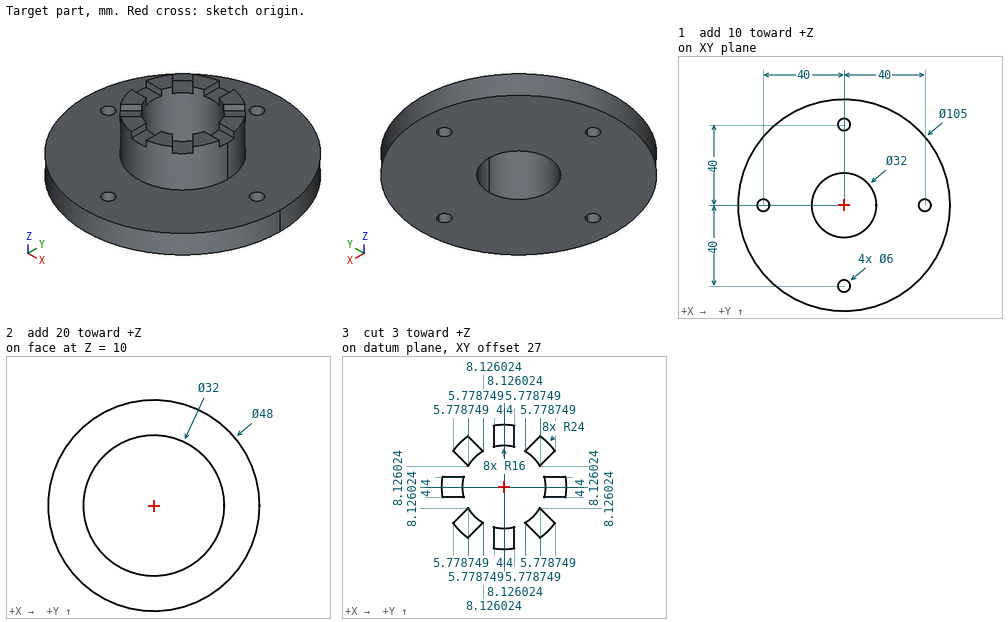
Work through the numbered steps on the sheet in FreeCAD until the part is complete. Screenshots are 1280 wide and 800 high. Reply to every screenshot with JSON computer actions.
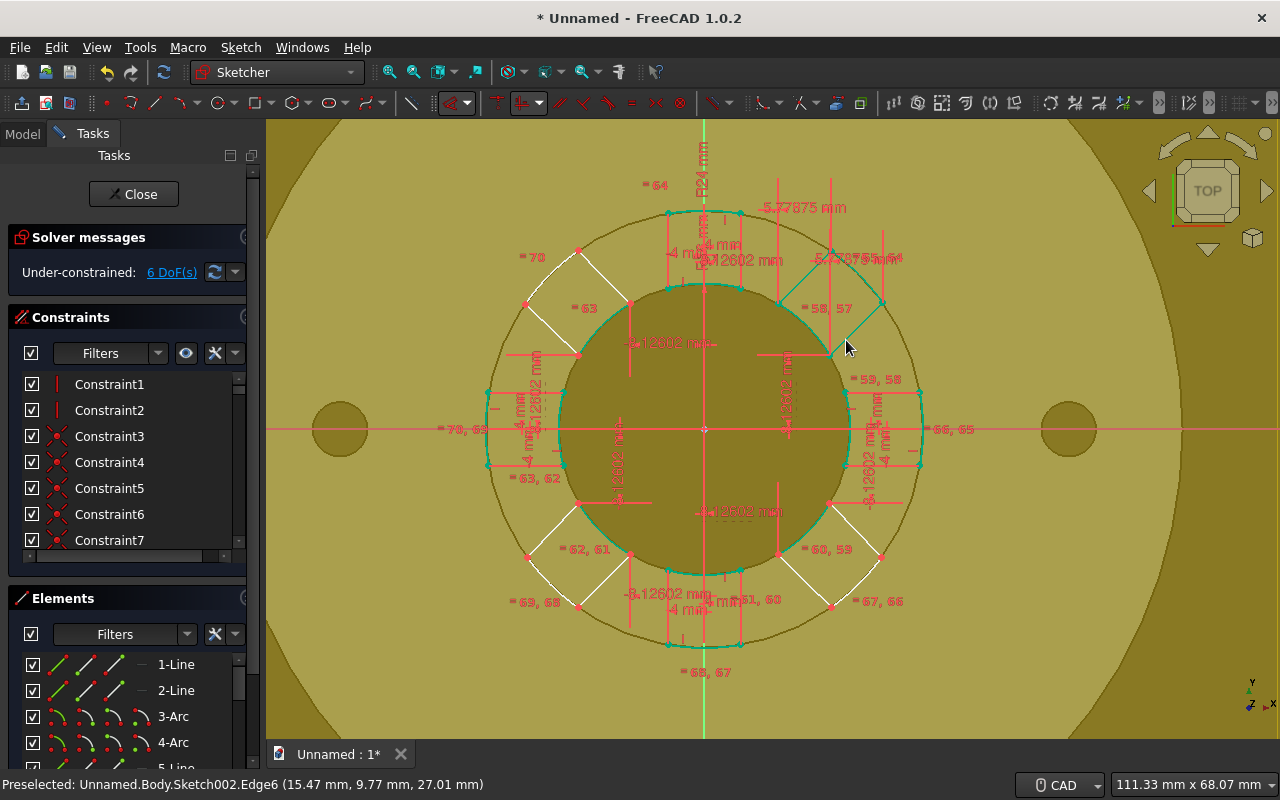
{"action": "left_click", "coordinate": [866, 541]}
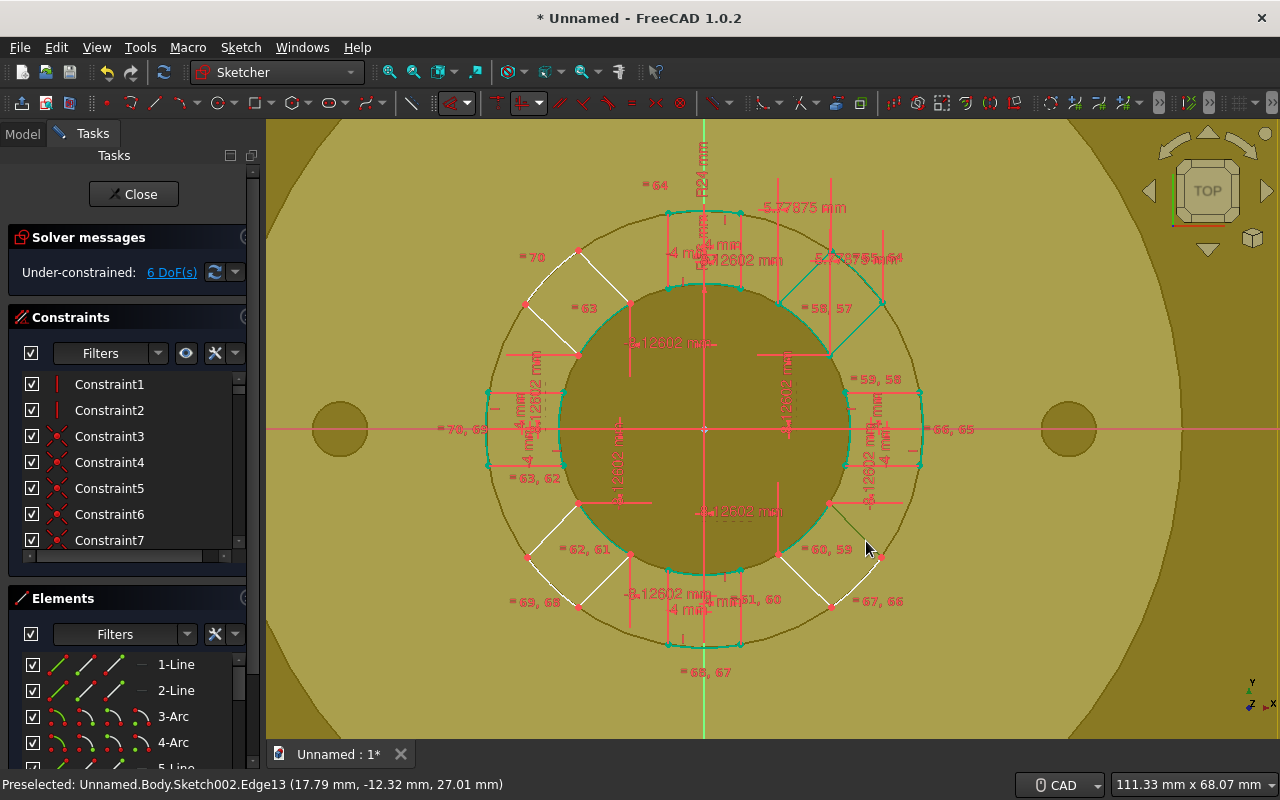
{"action": "key", "text": "l"}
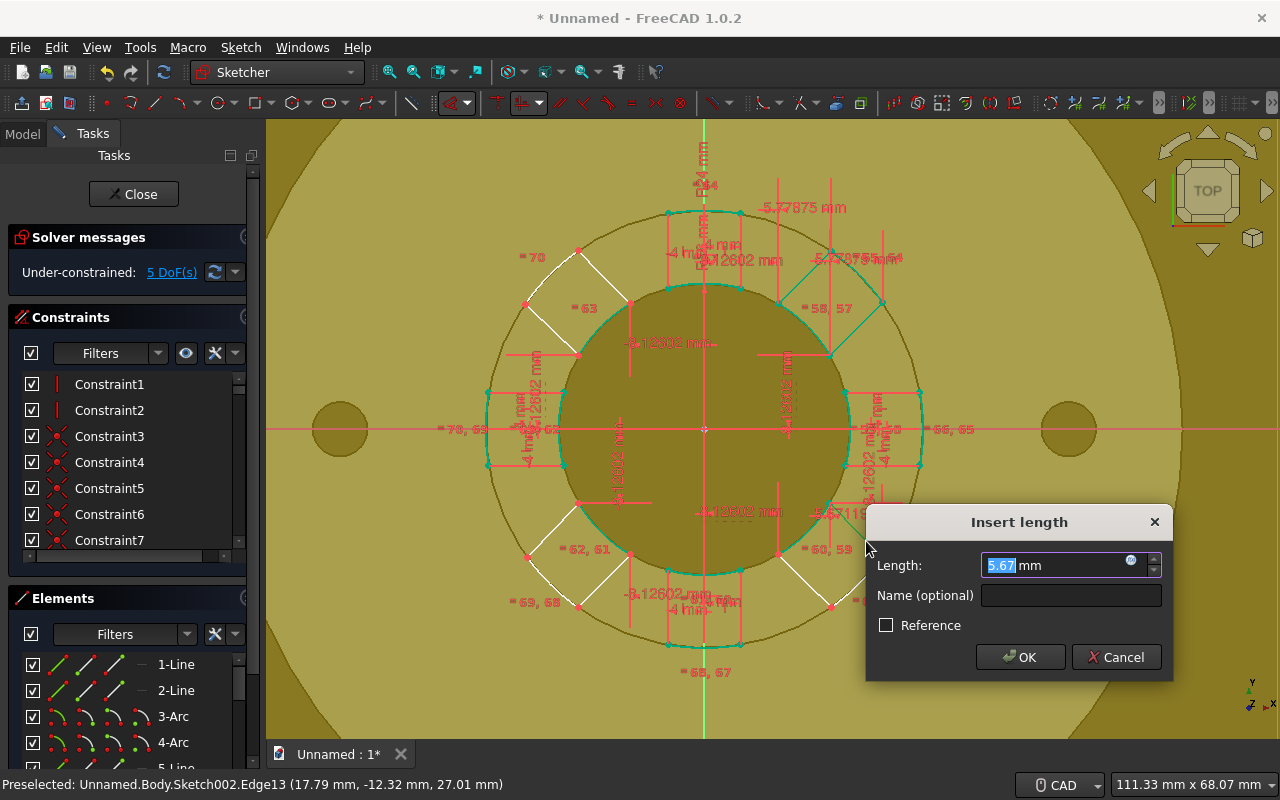
{"action": "type", "text": "5.778749"}
{"action": "key", "text": "Return"}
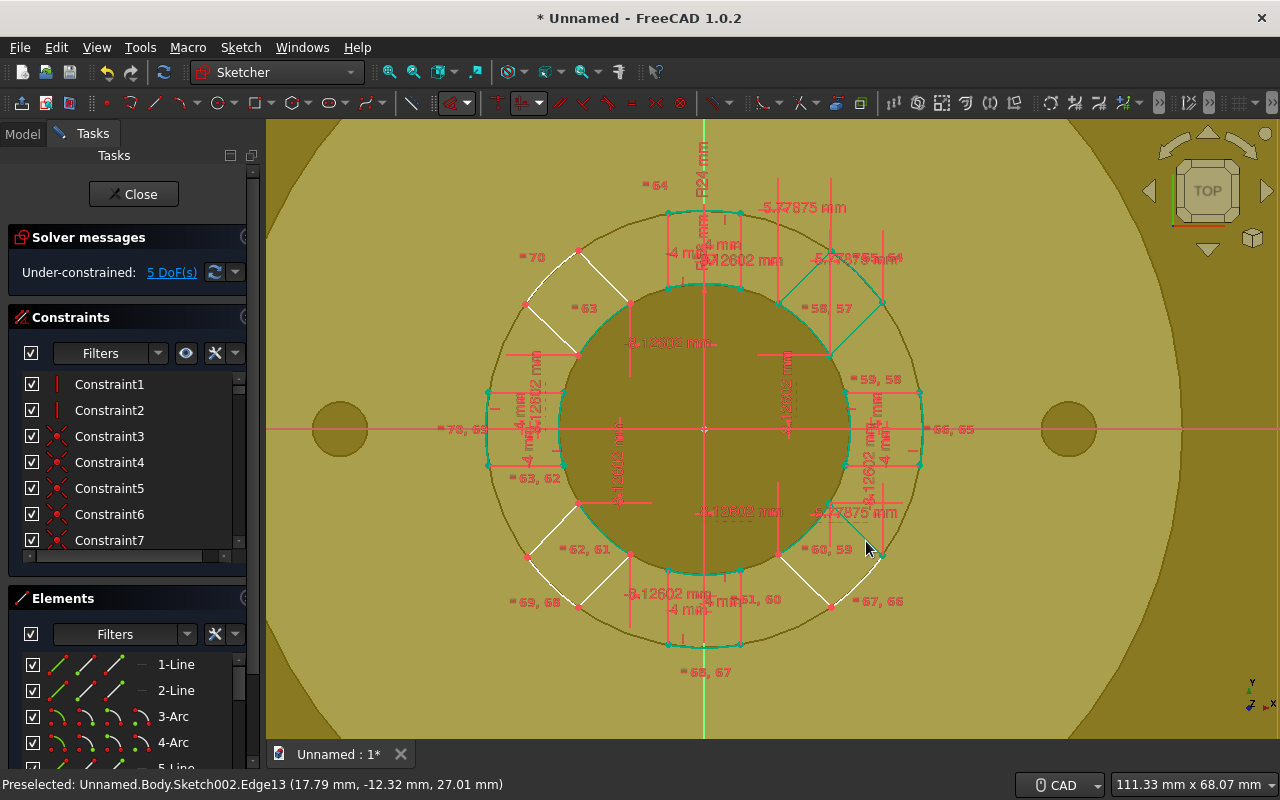
{"action": "left_click", "coordinate": [794, 571]}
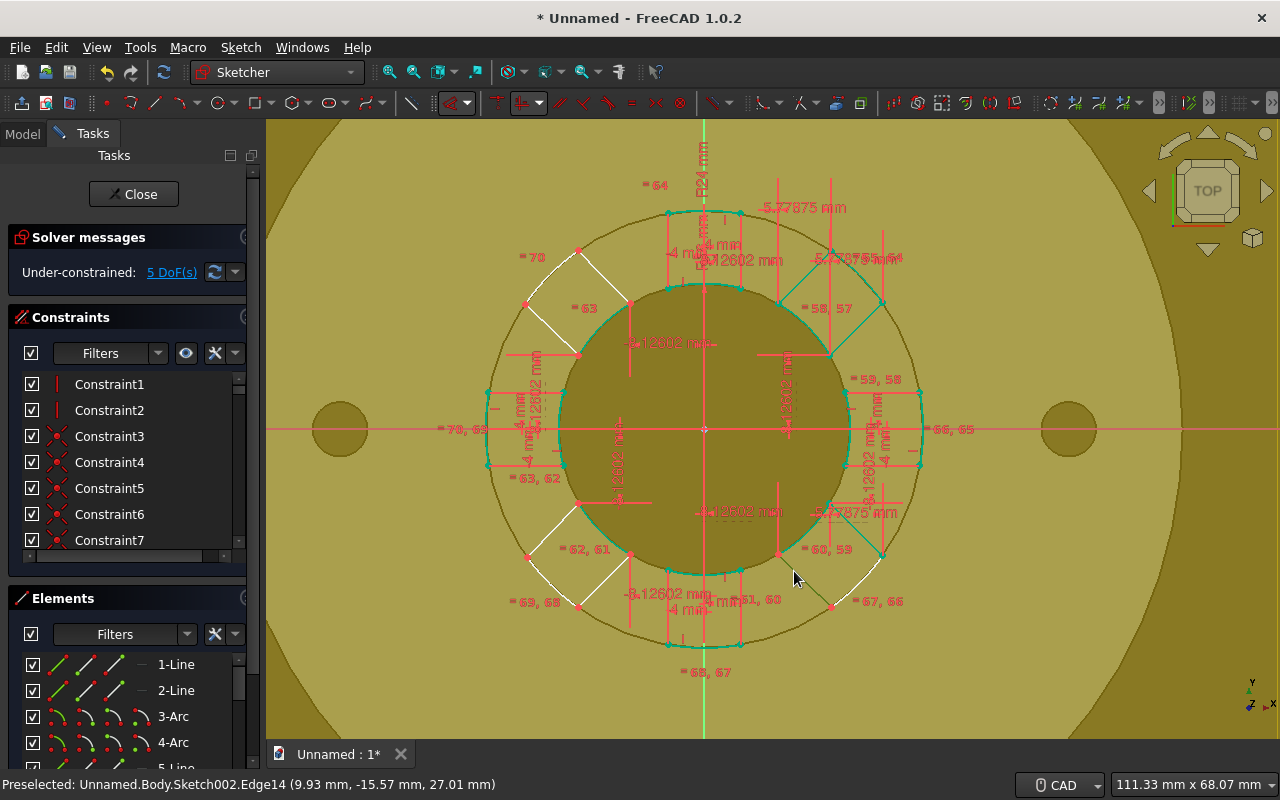
{"action": "left_click", "coordinate": [470, 104]}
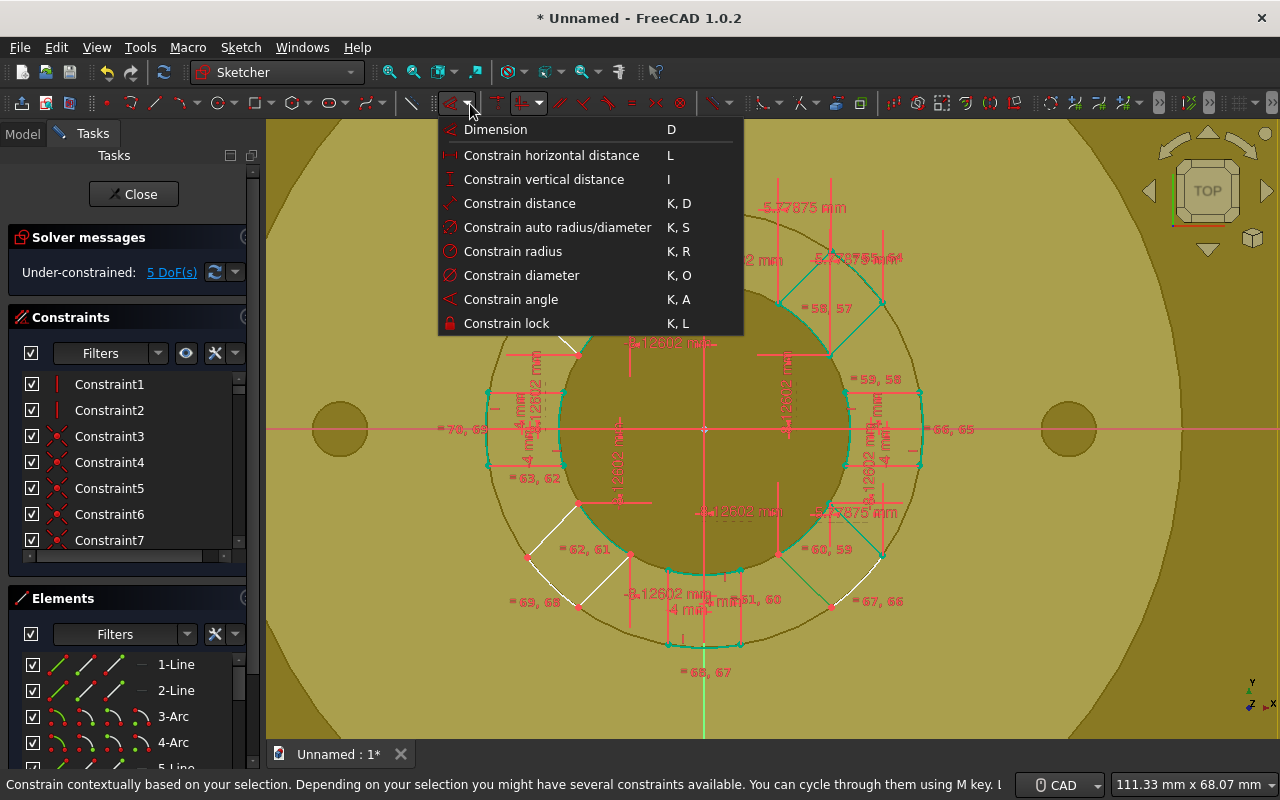
{"action": "left_click", "coordinate": [591, 155]}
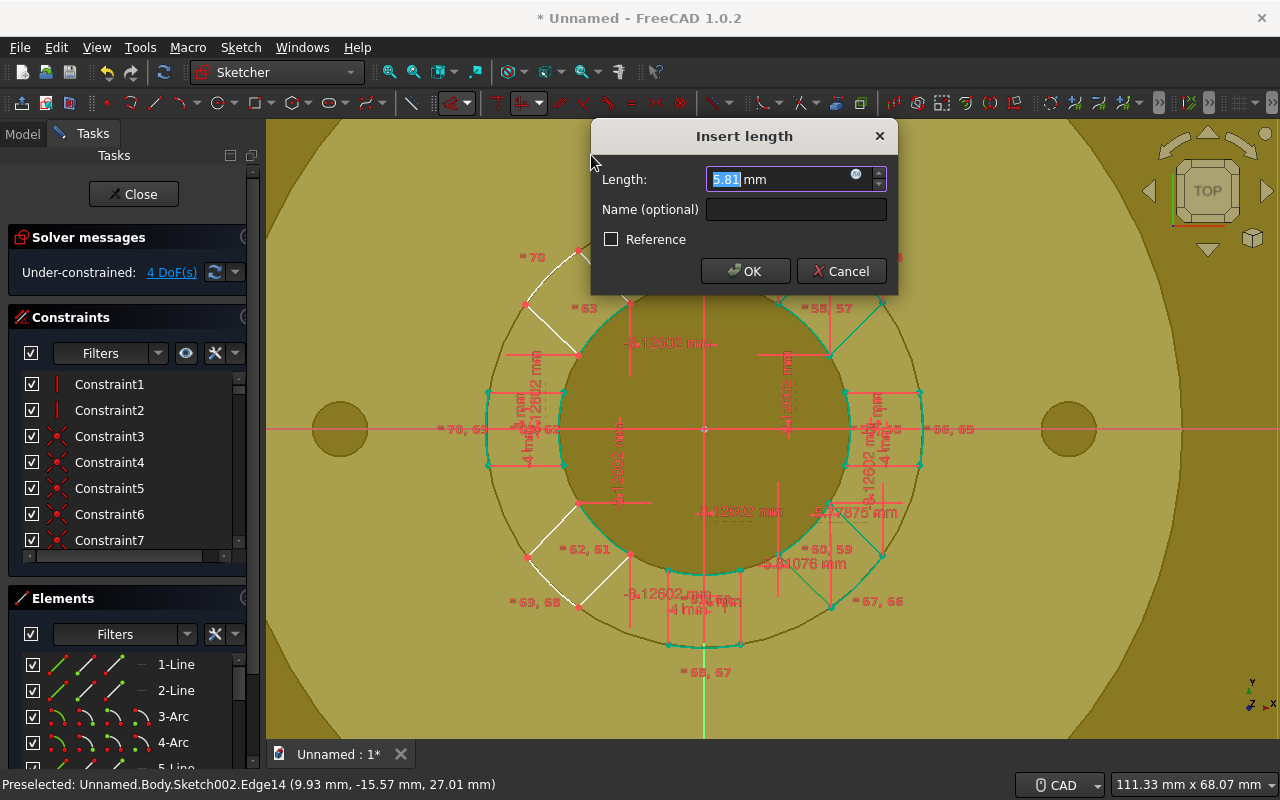
{"action": "type", "text": "5.778749"}
{"action": "key", "text": "Return"}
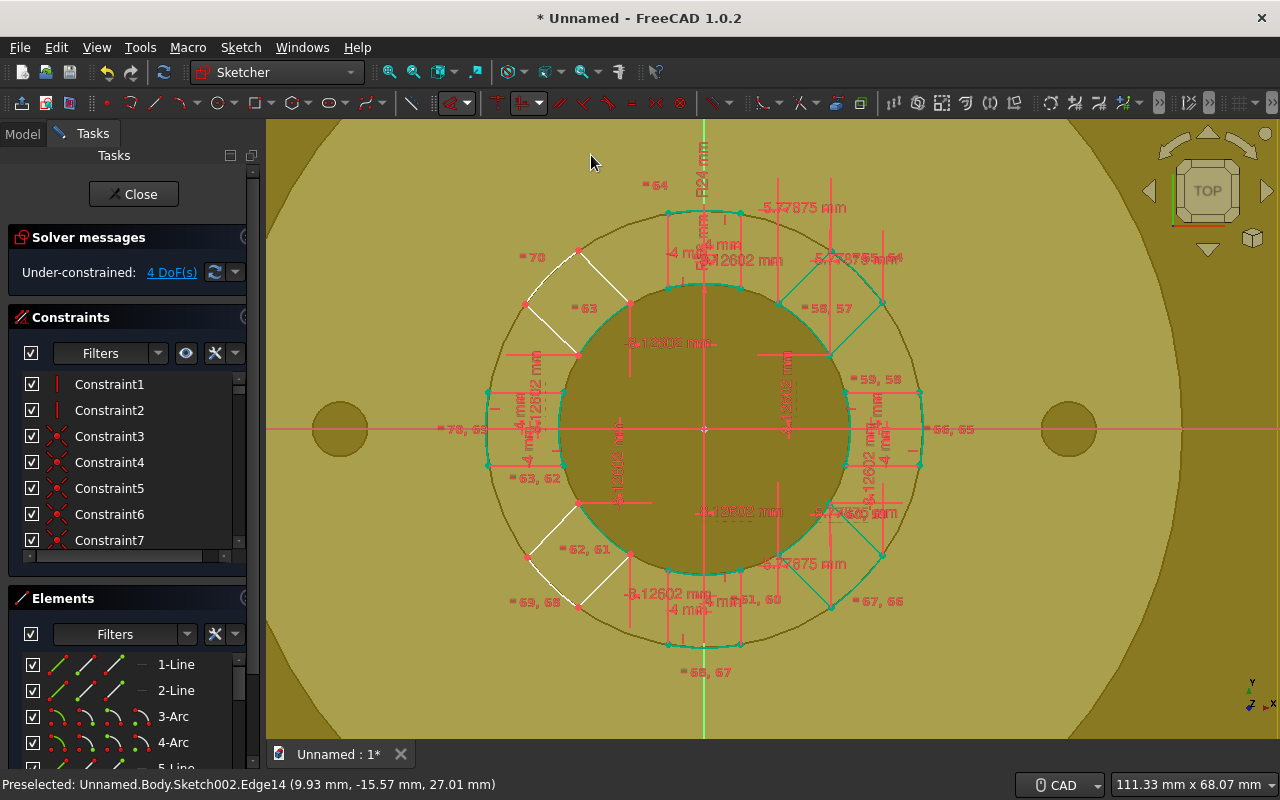
{"action": "left_click", "coordinate": [594, 592]}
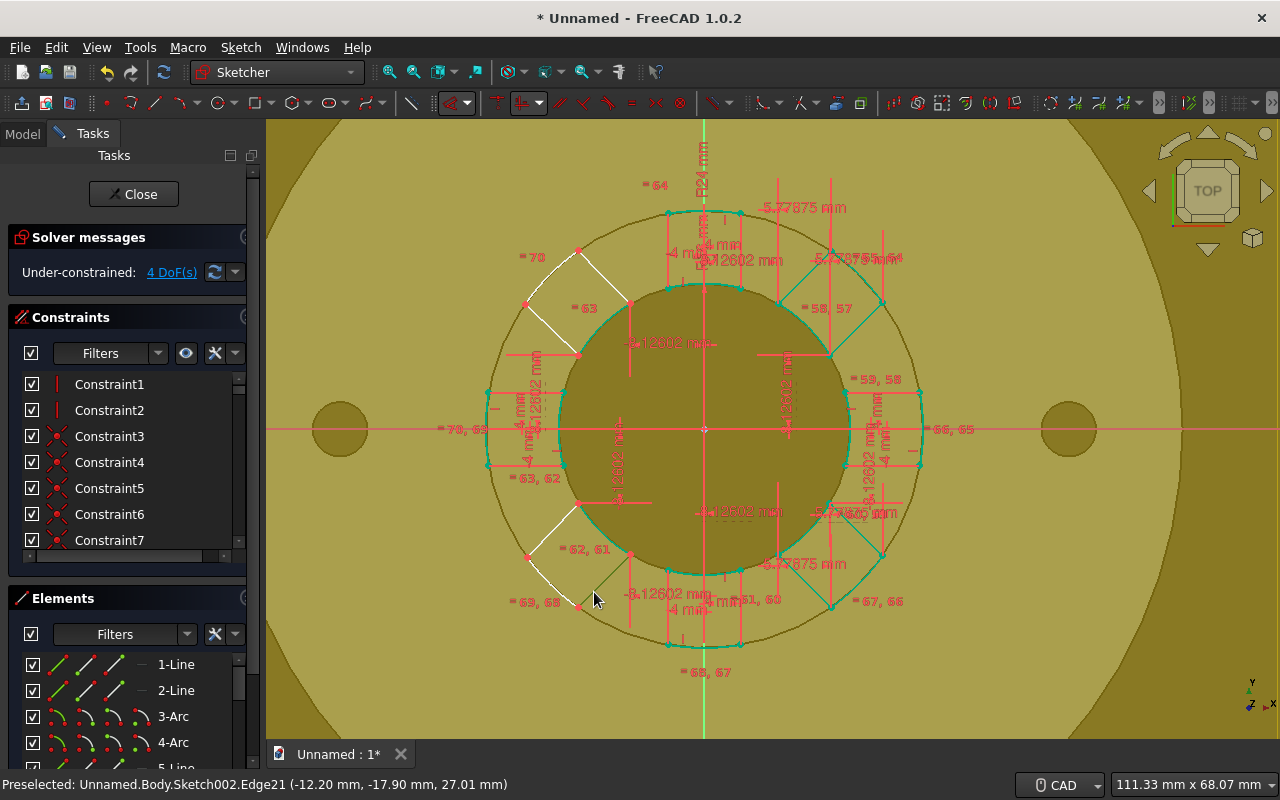
{"action": "left_click", "coordinate": [470, 104]}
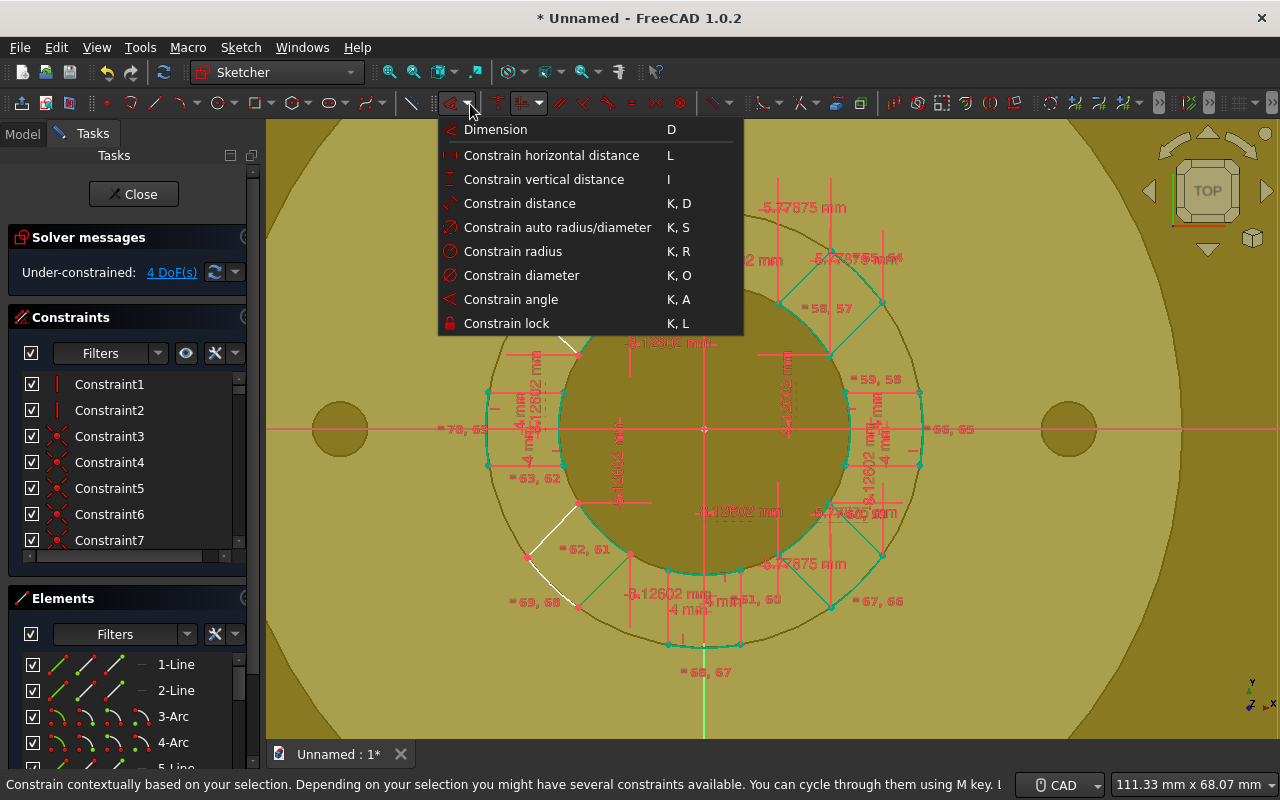
{"action": "left_click", "coordinate": [591, 155]}